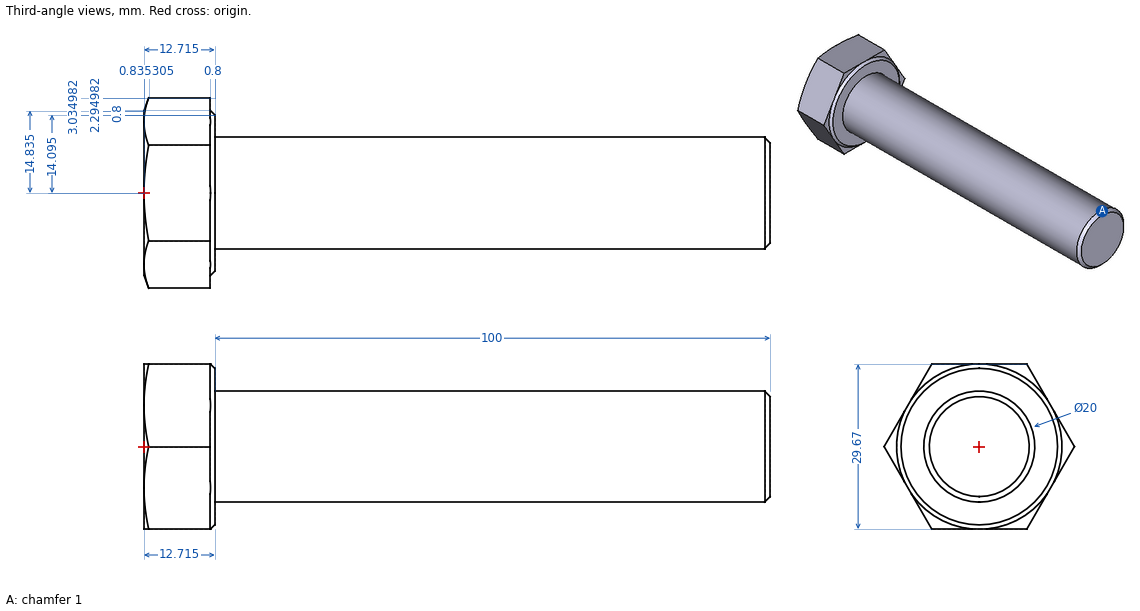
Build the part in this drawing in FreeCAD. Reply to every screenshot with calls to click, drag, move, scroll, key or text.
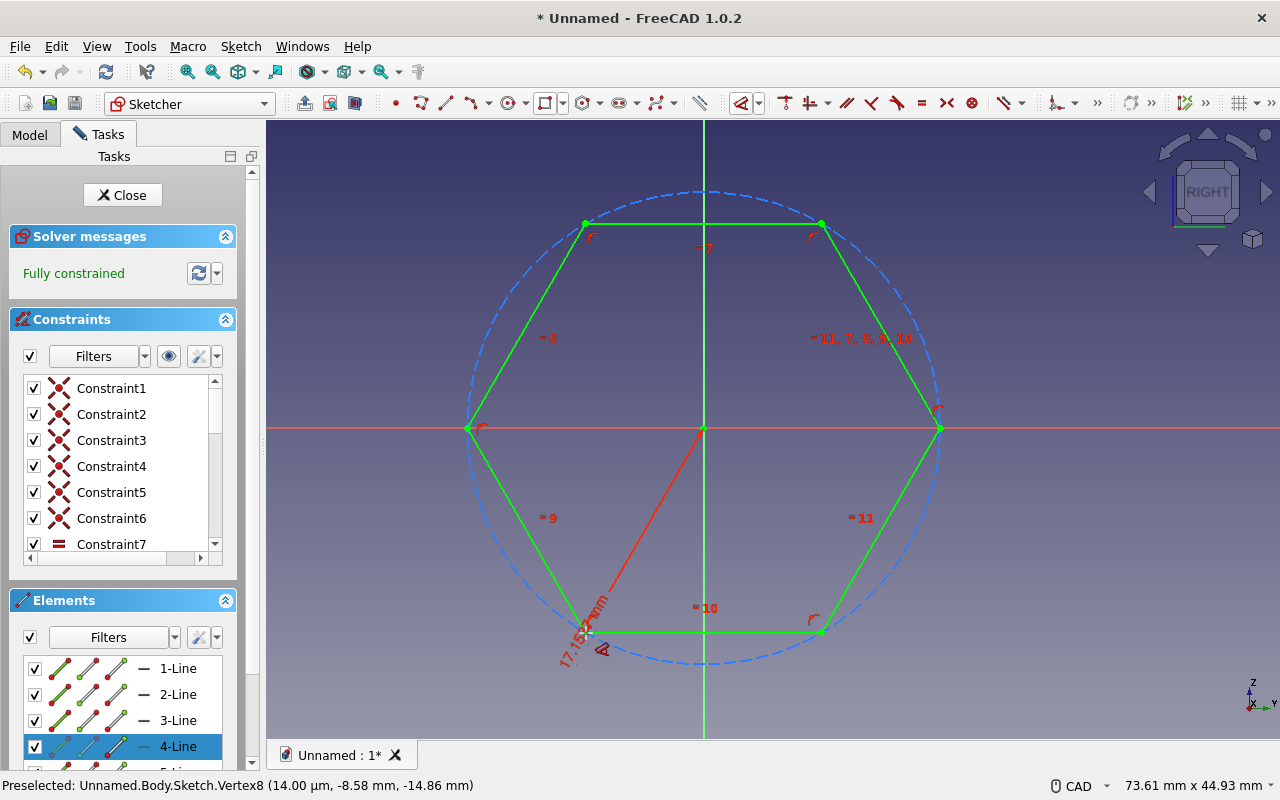
click(822, 224)
click(856, 334)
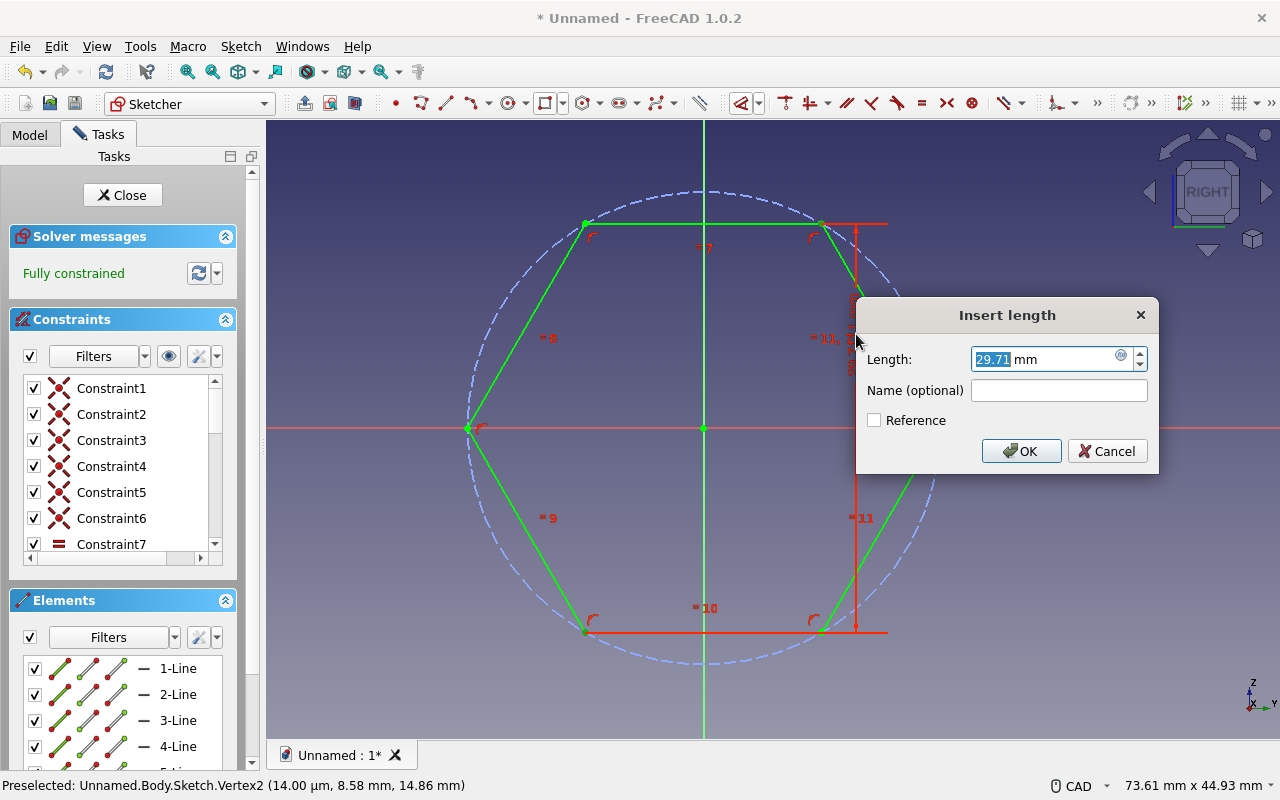
text(29.67)
key(Return)
key(Escape)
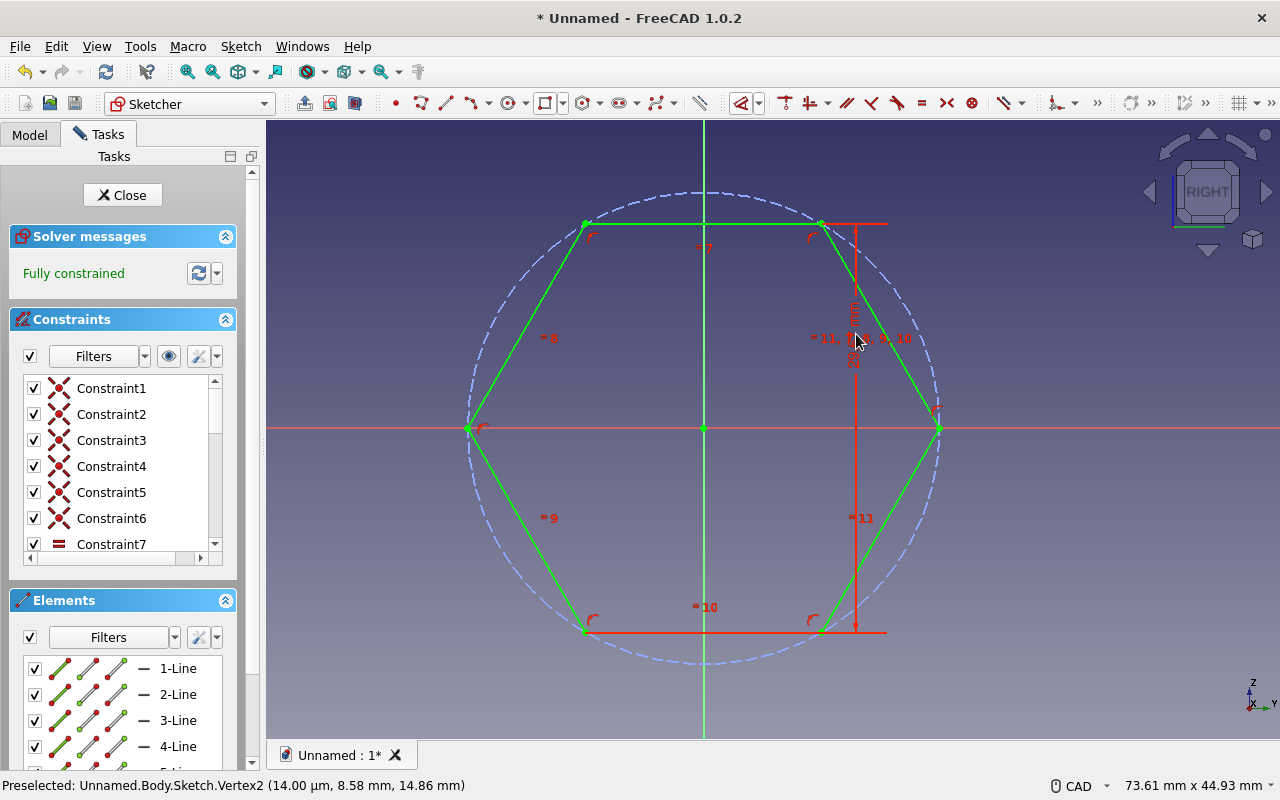
click(123, 195)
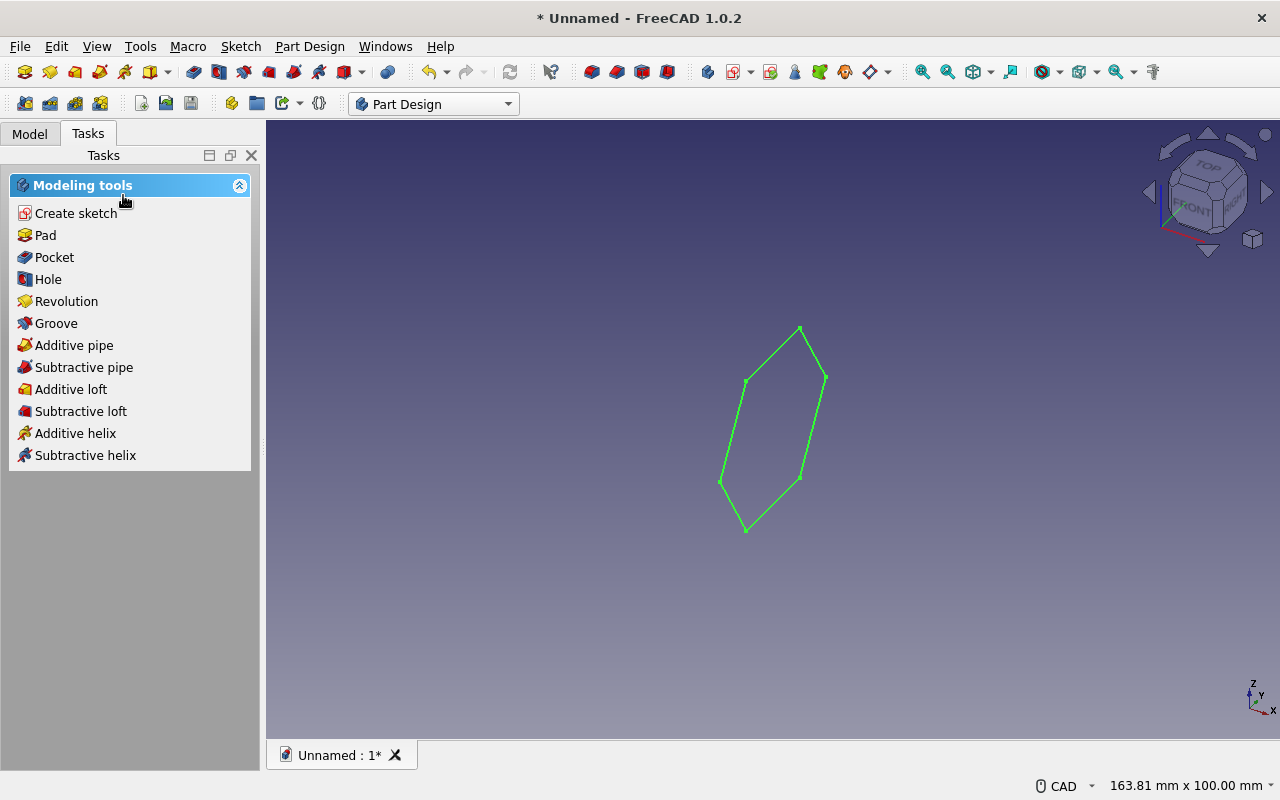
click(25, 72)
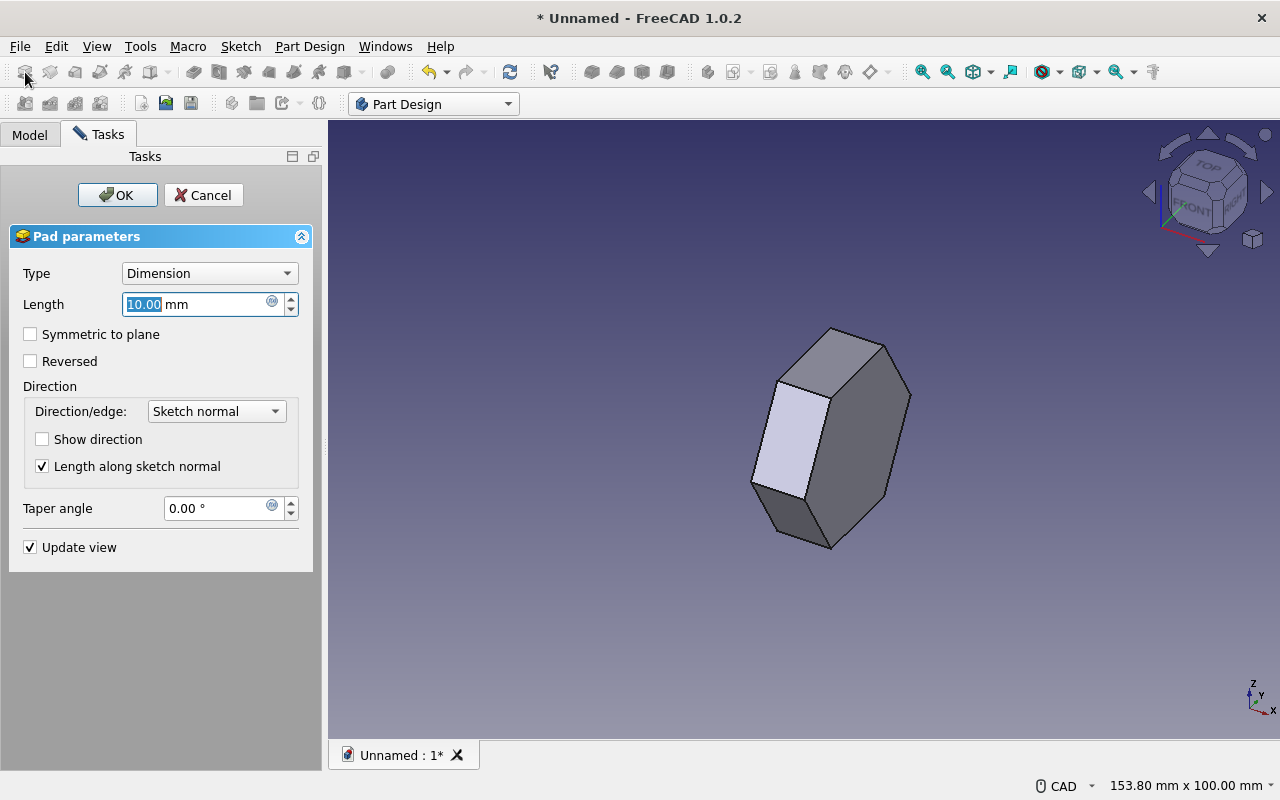
text(12.715)
key(Tab)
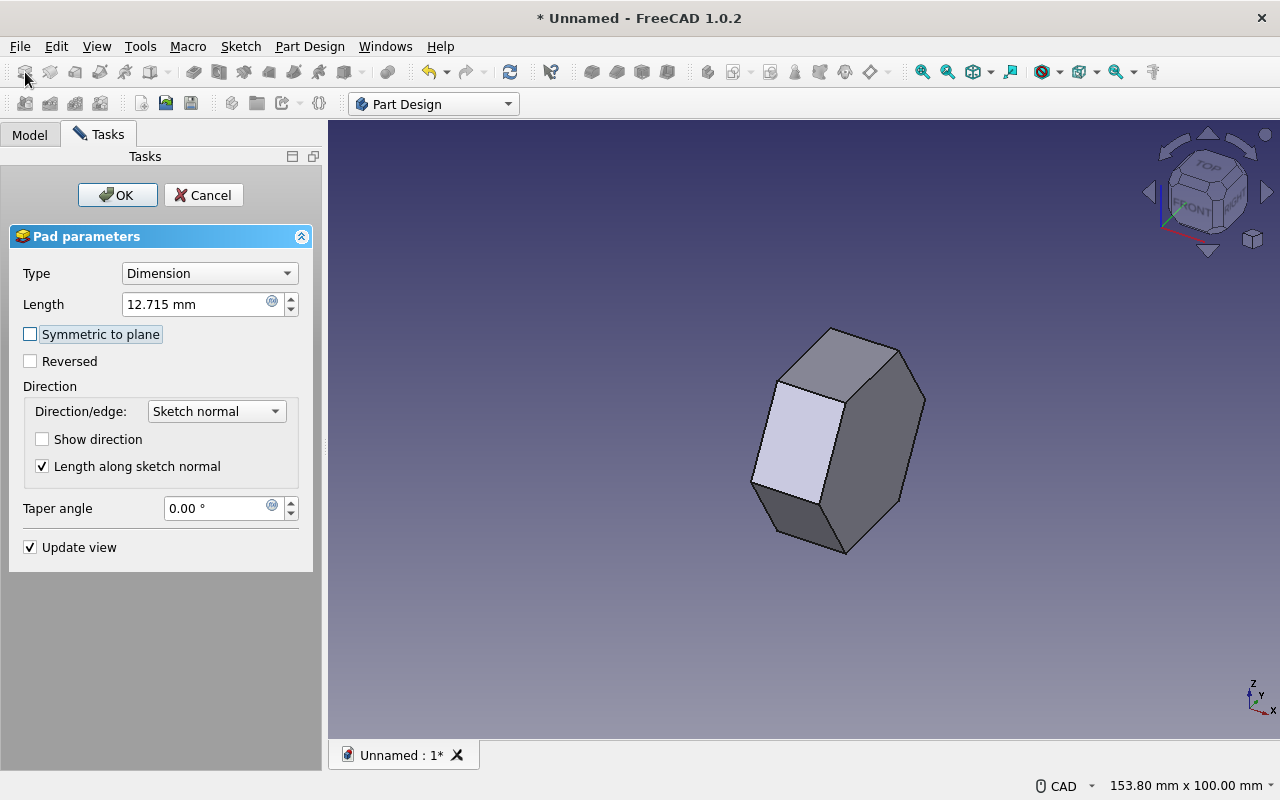
click(118, 195)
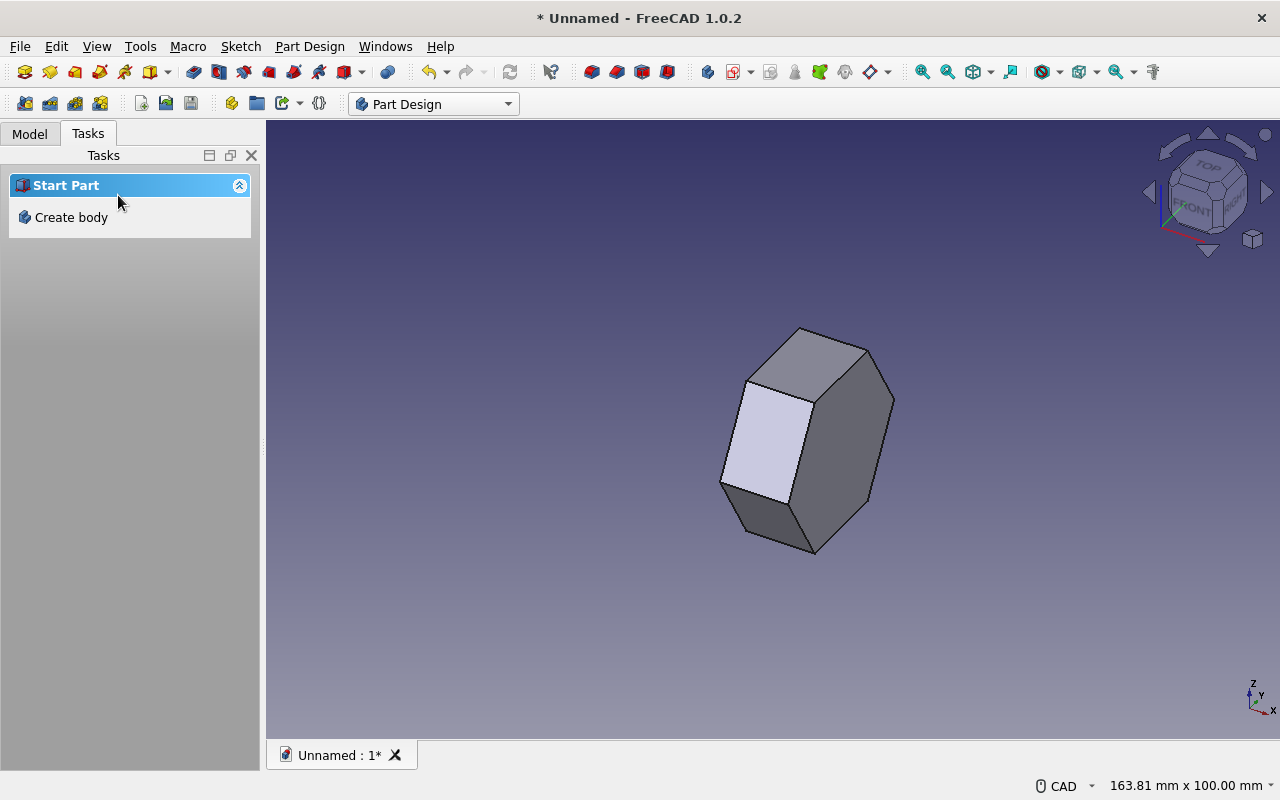
key(v)
key(f)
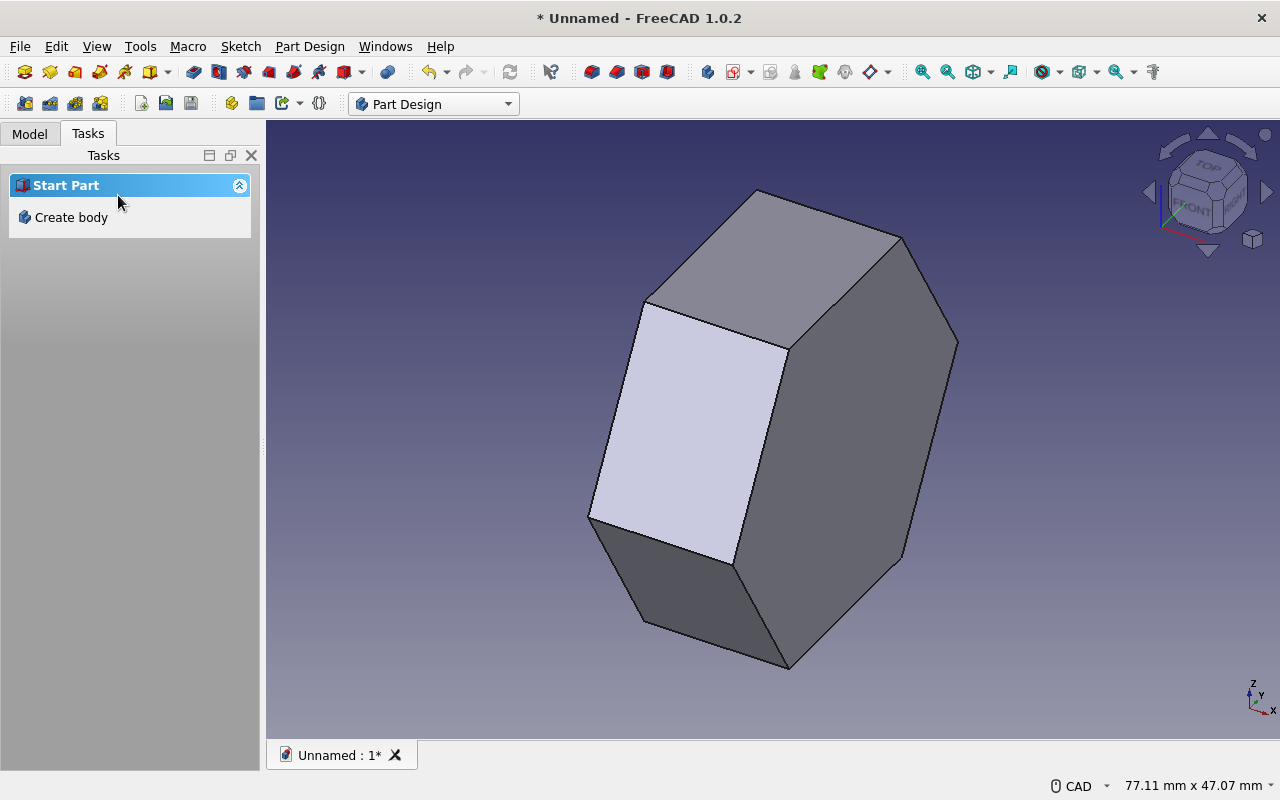
click(732, 72)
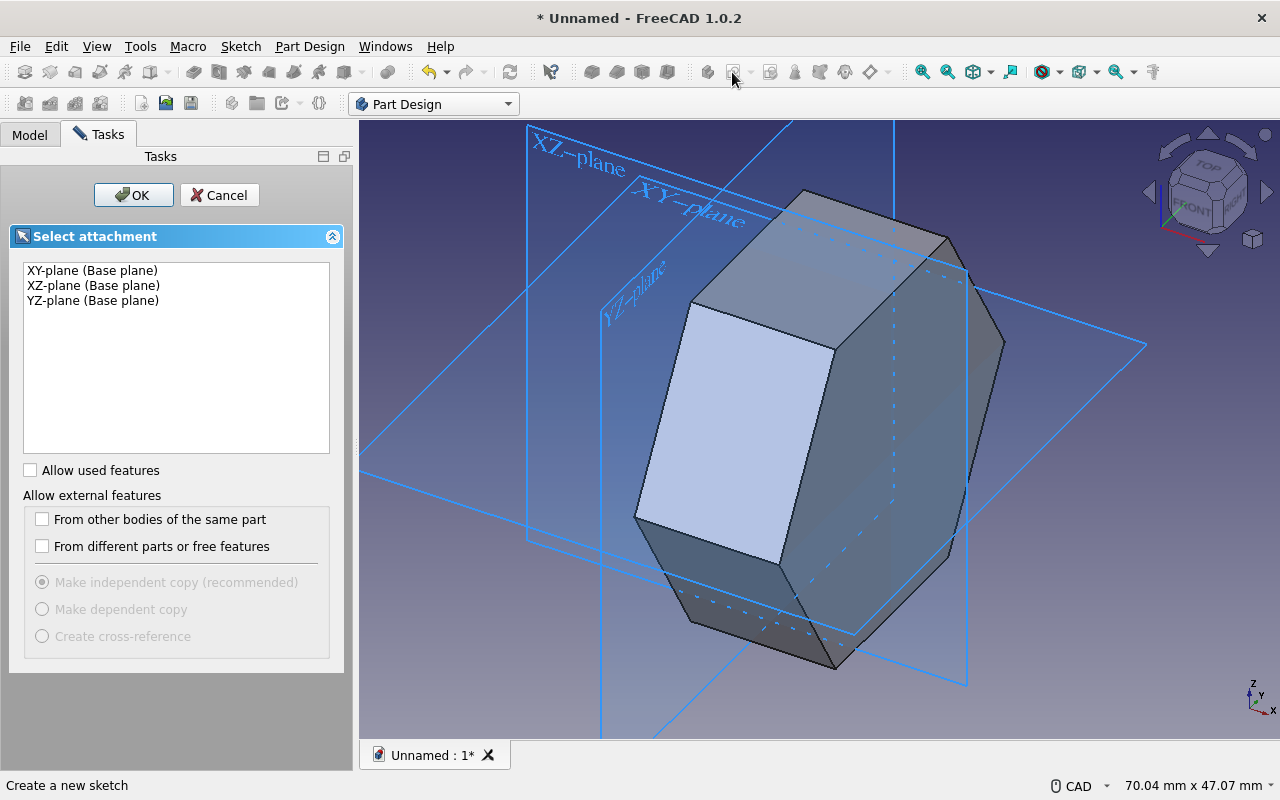
click(84, 270)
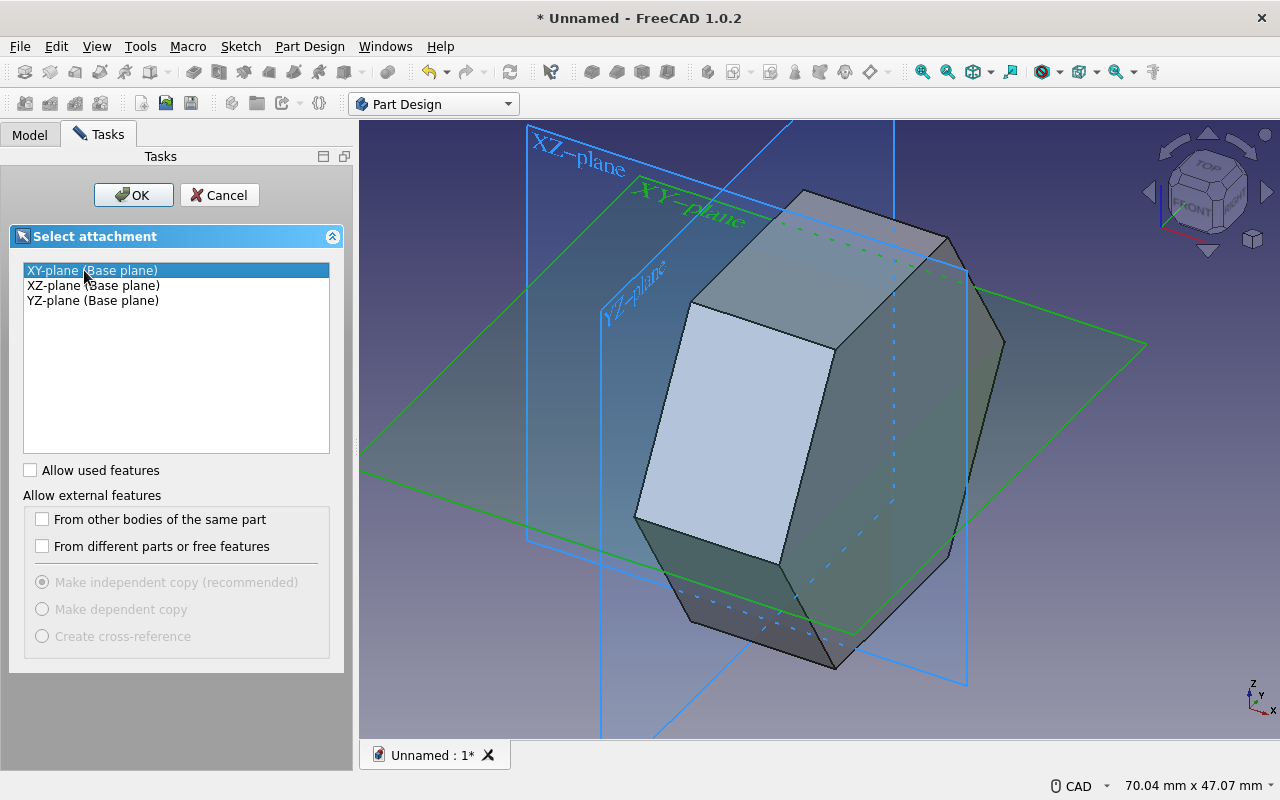
click(134, 195)